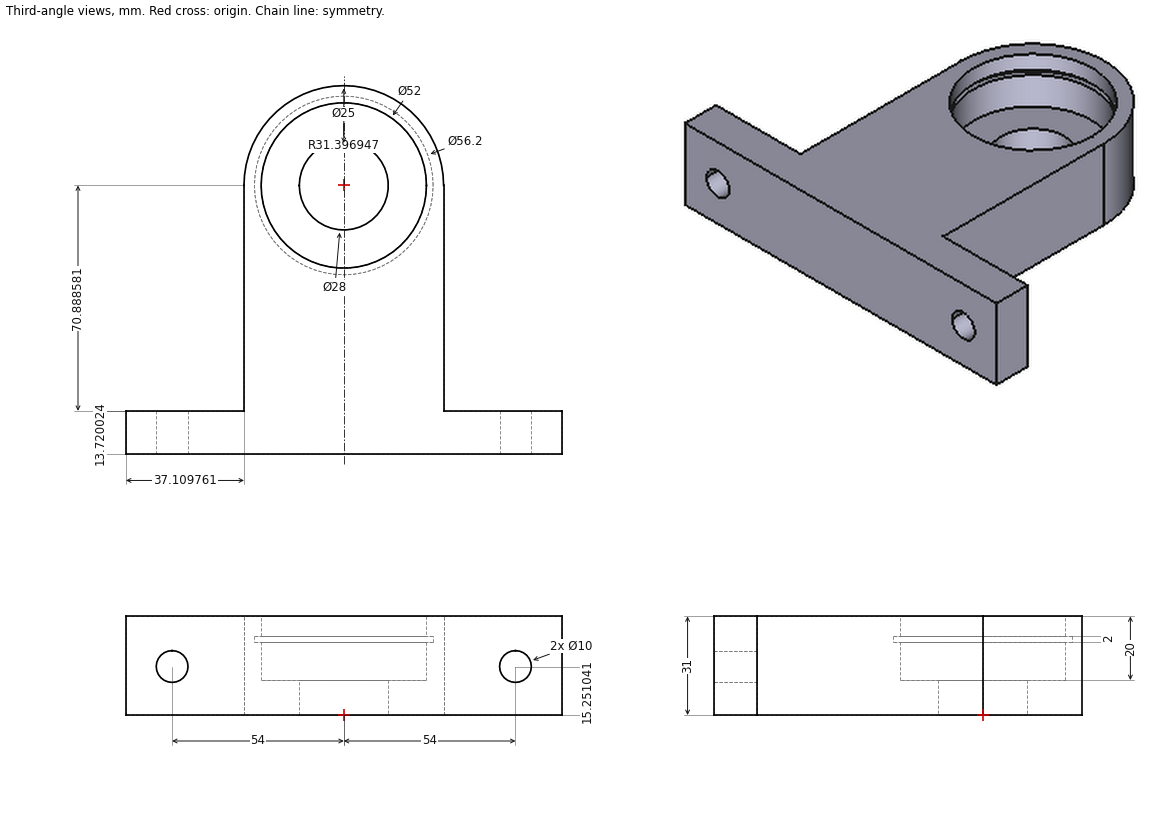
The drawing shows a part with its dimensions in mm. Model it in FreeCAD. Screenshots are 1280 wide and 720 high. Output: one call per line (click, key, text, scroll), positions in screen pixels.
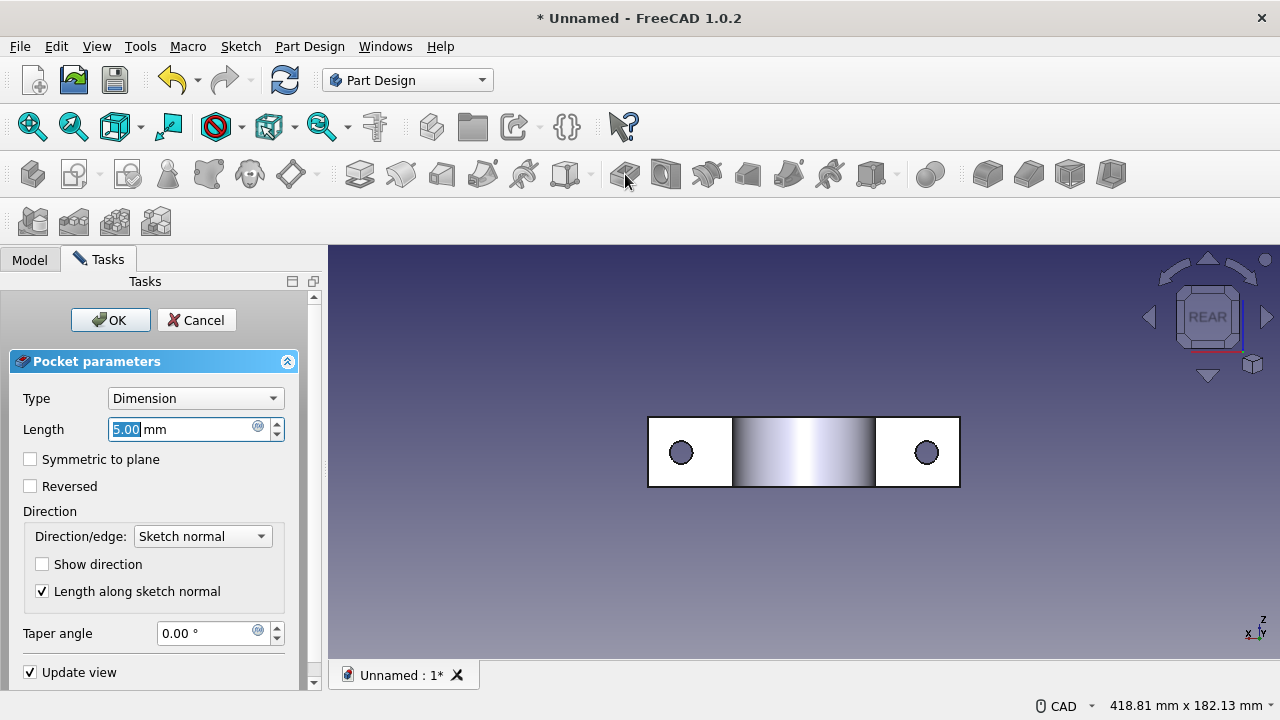
click(196, 398)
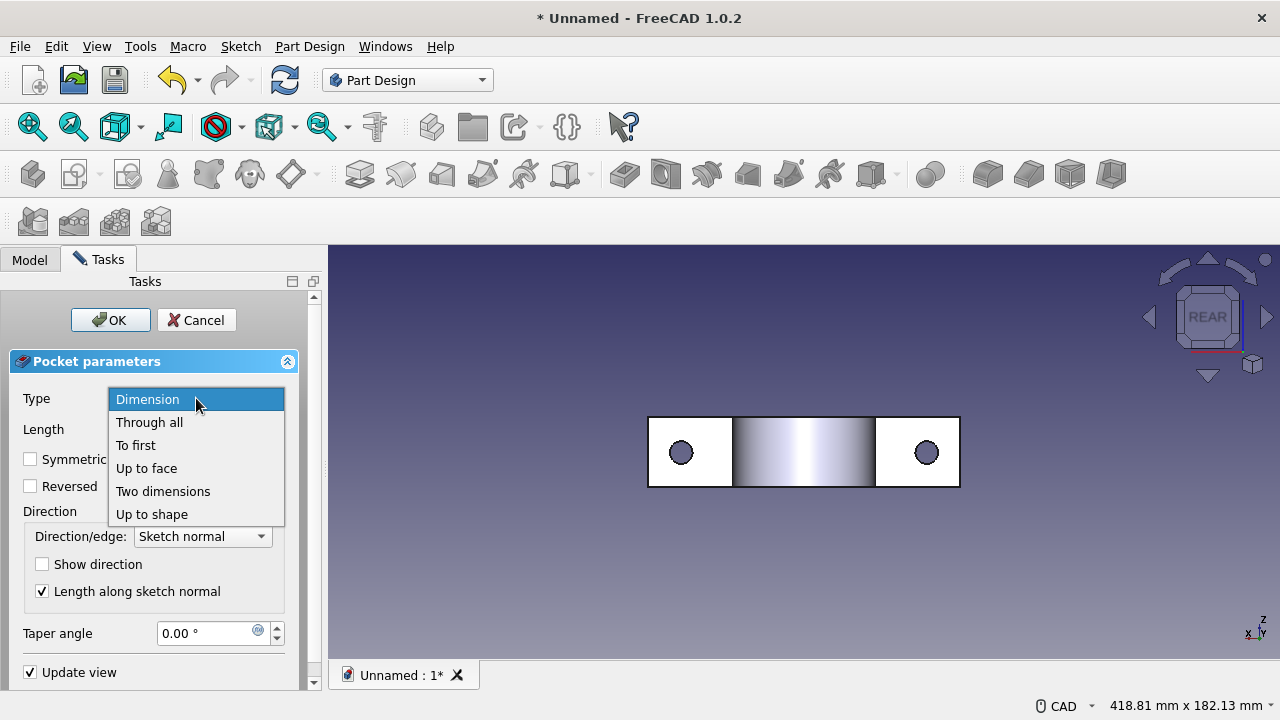
click(194, 422)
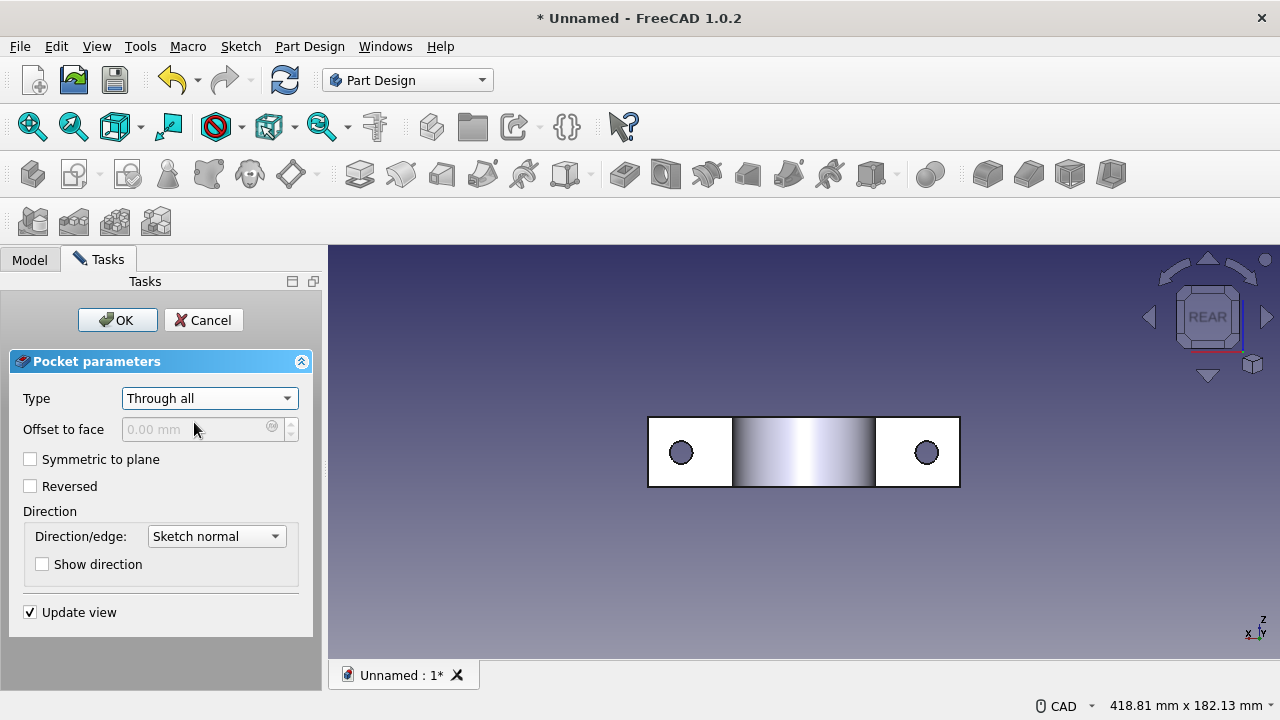
click(31, 486)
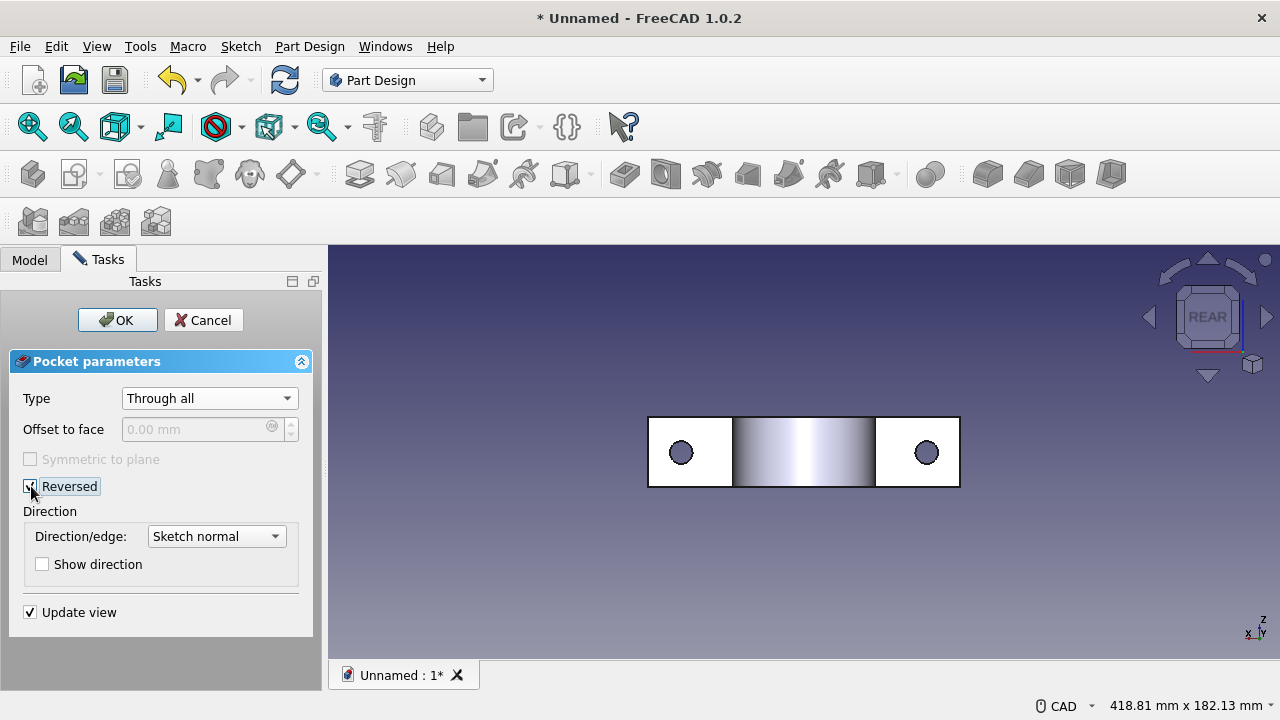
click(118, 320)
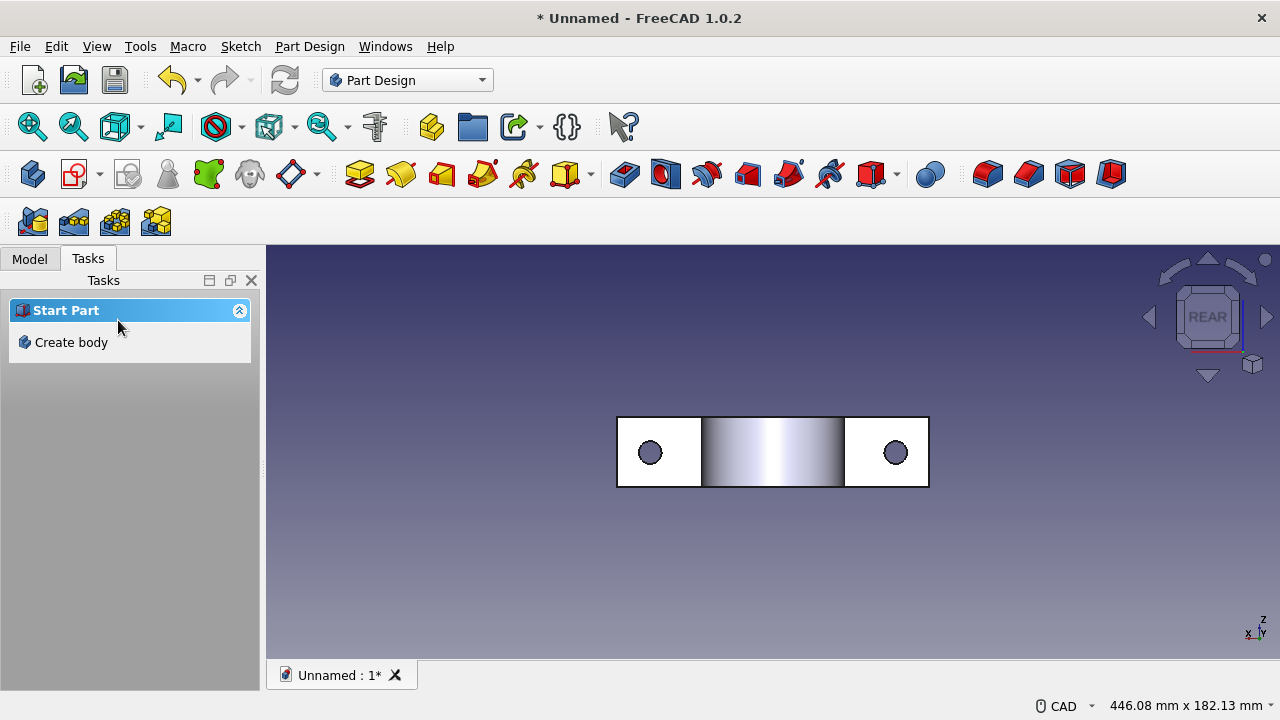
key(v)
key(f)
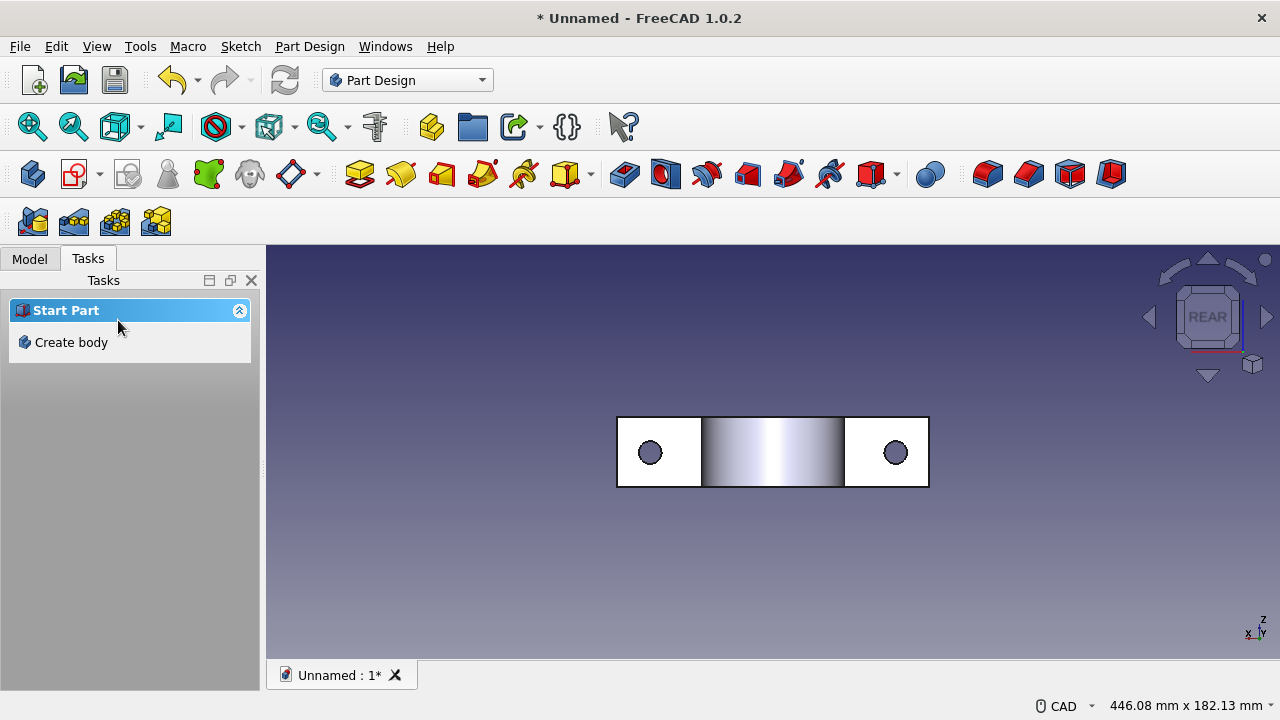
key(0)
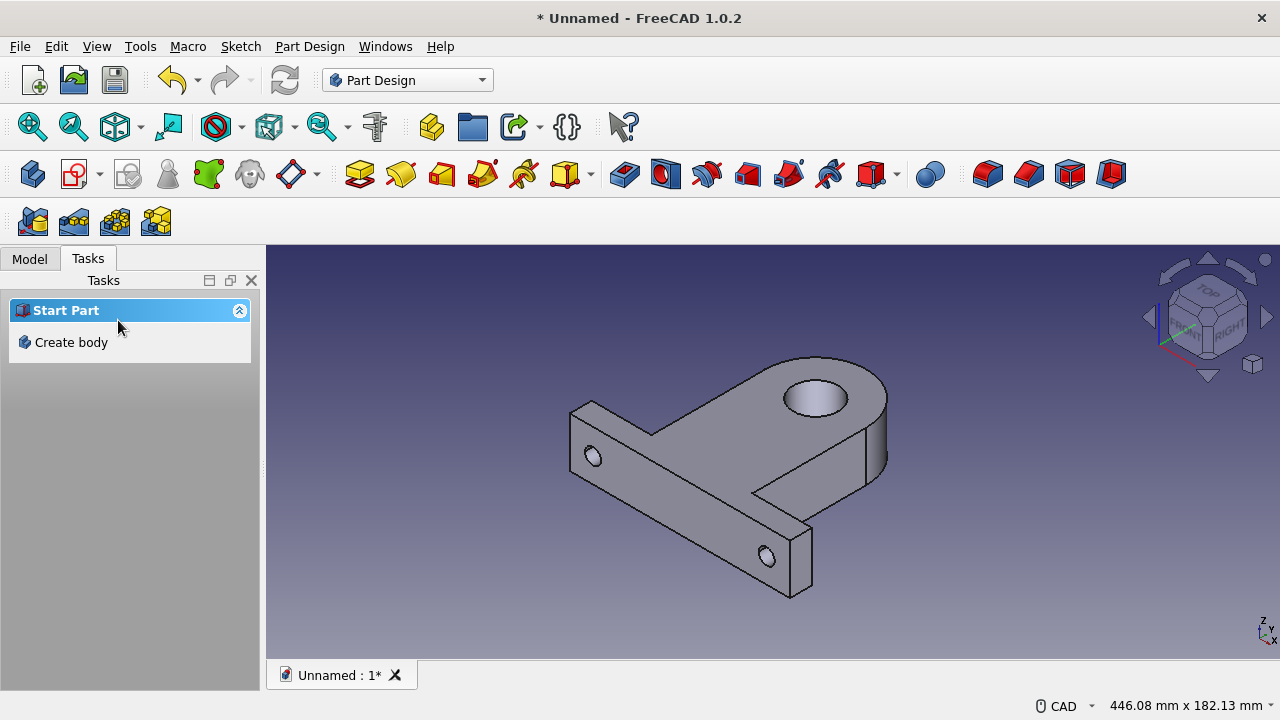
click(746, 438)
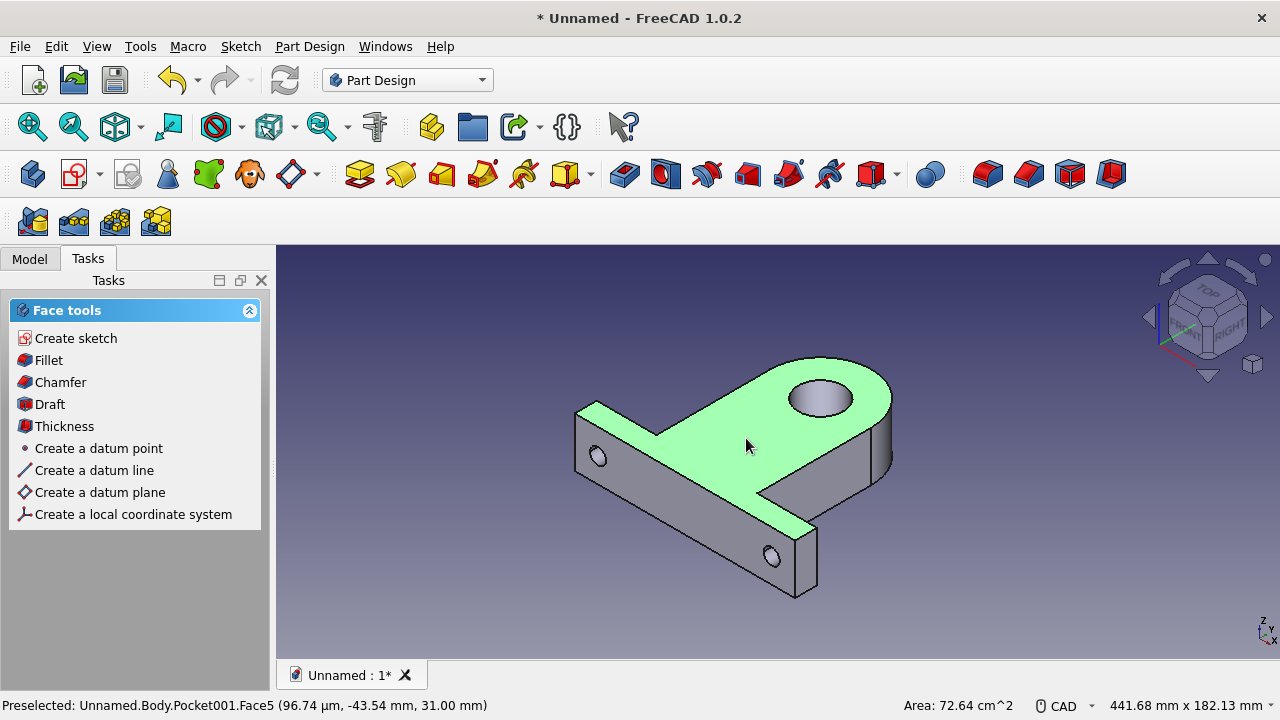
click(74, 174)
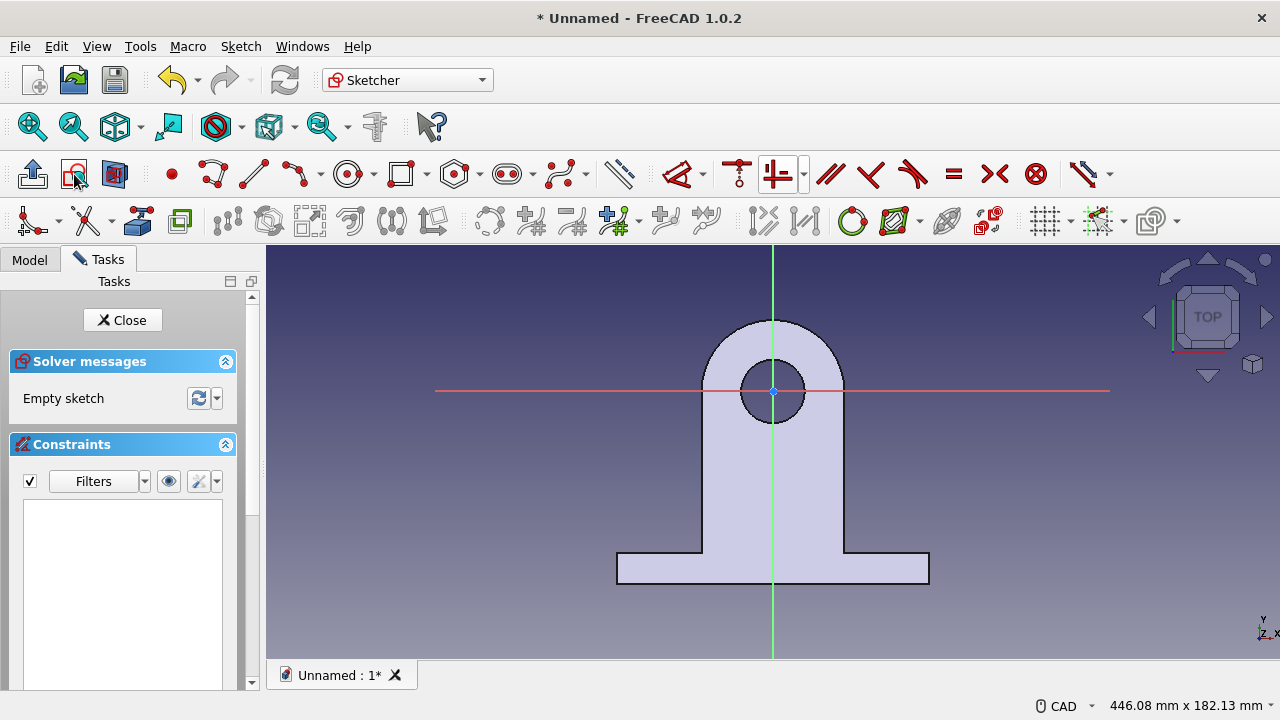
scroll(829, 342, up, 4)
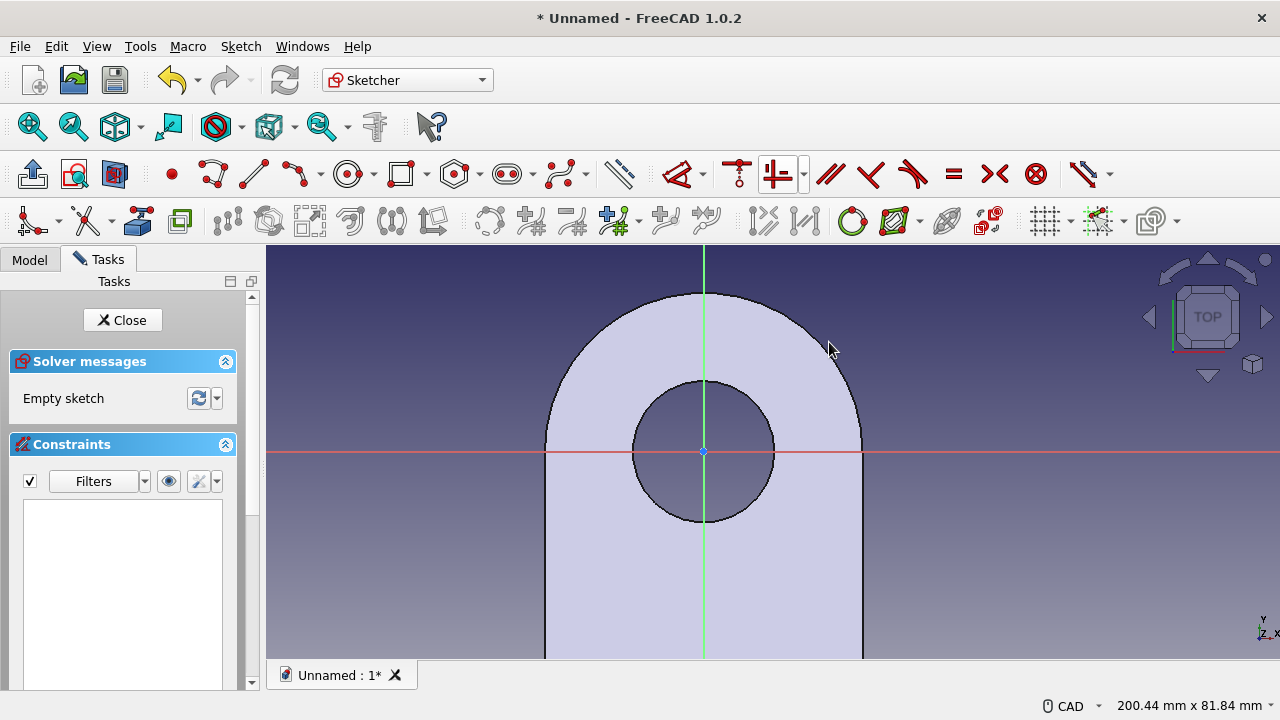
click(348, 174)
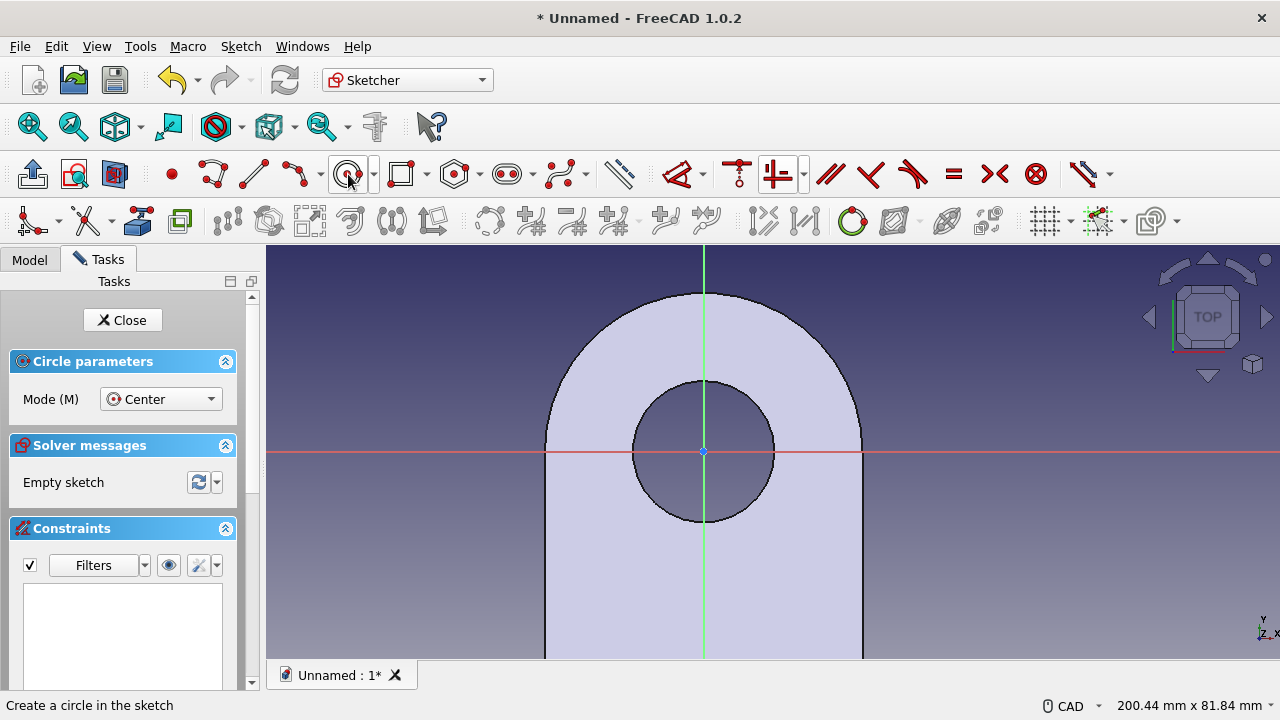
click(704, 452)
click(797, 359)
key(Escape)